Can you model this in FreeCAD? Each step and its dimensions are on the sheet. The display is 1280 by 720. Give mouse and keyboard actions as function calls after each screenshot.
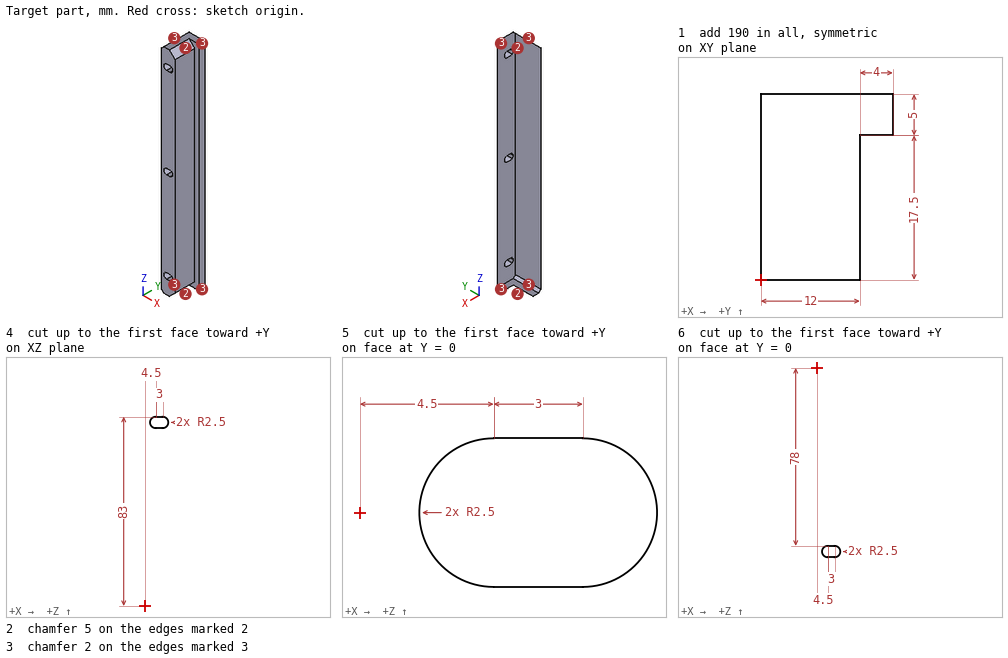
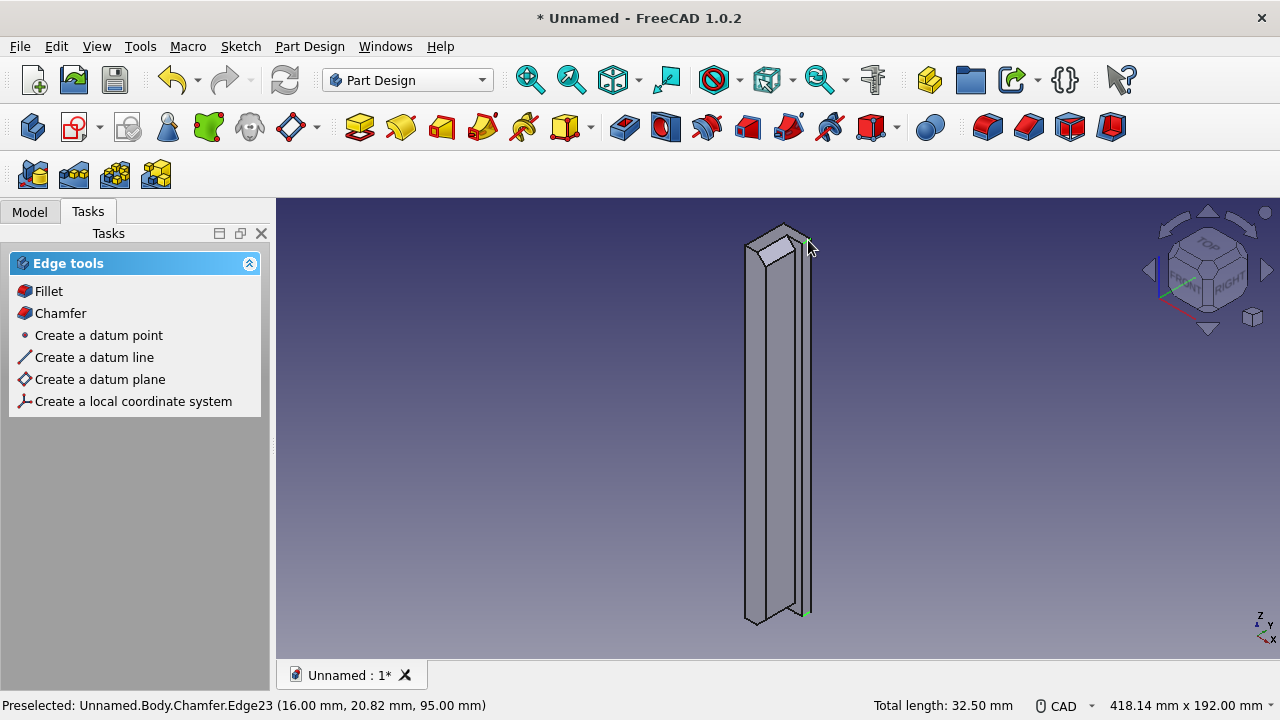
key(2)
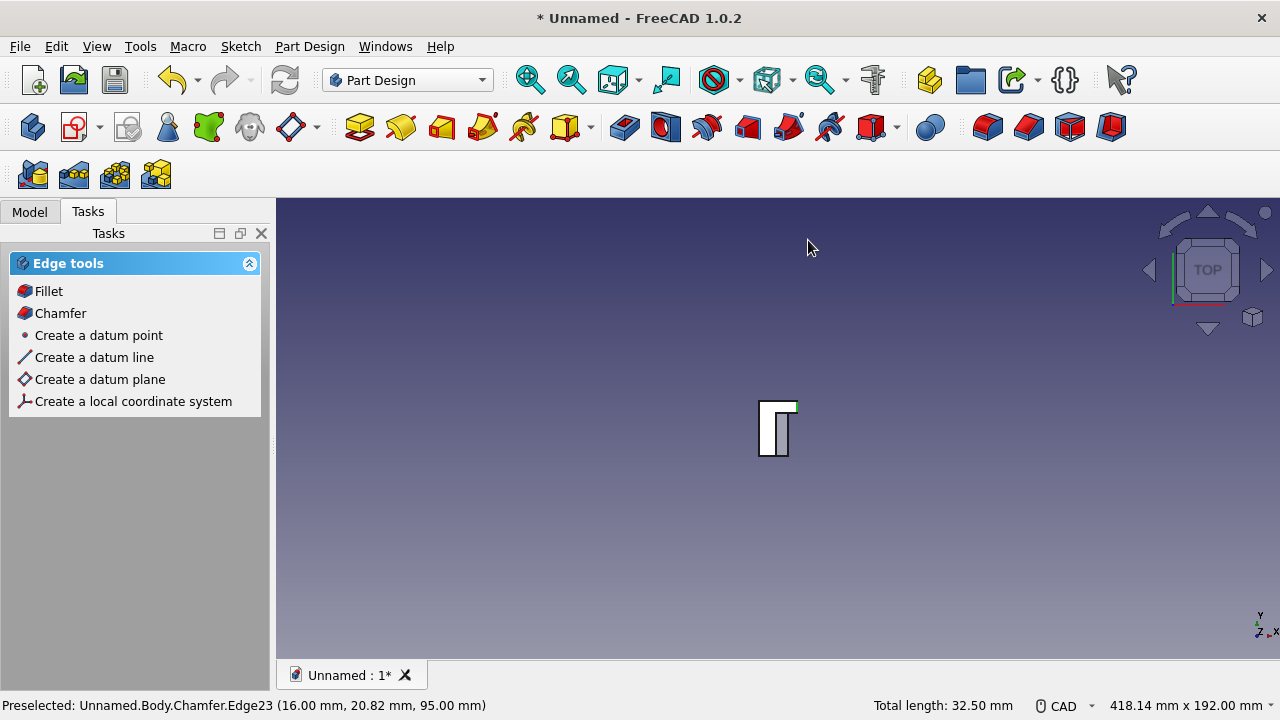
click(531, 80)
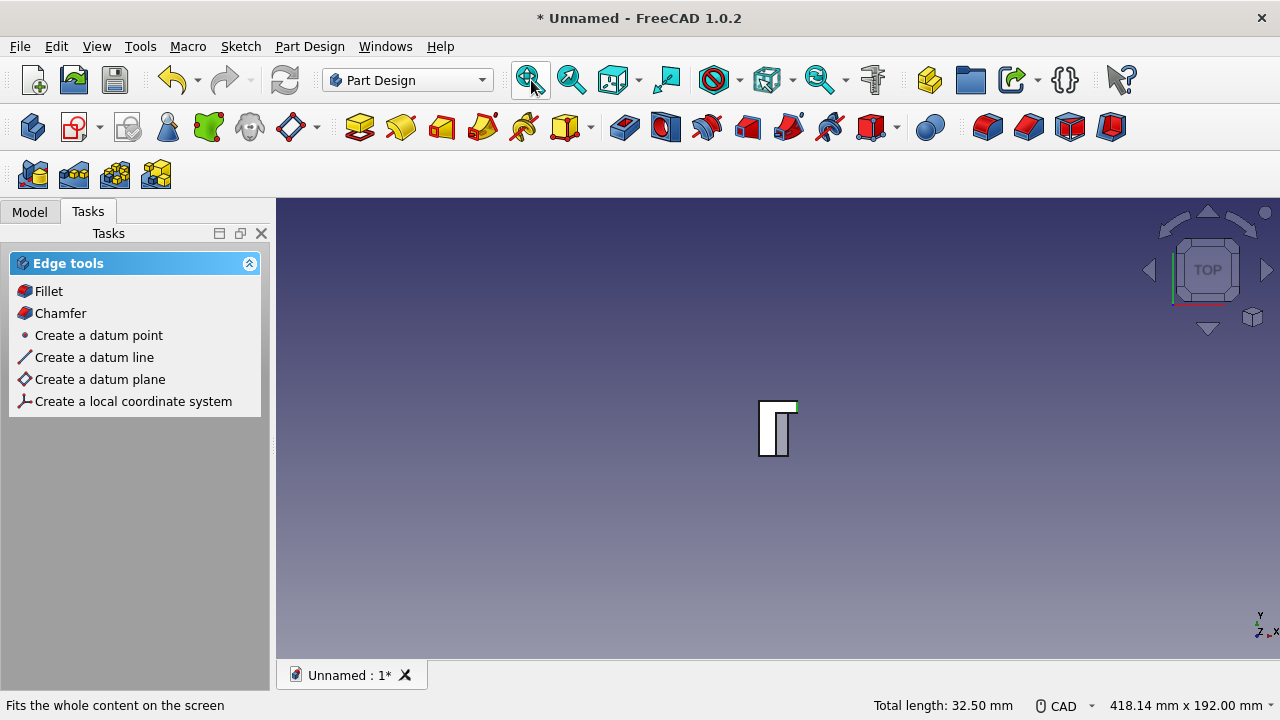
click(759, 427, ctrl)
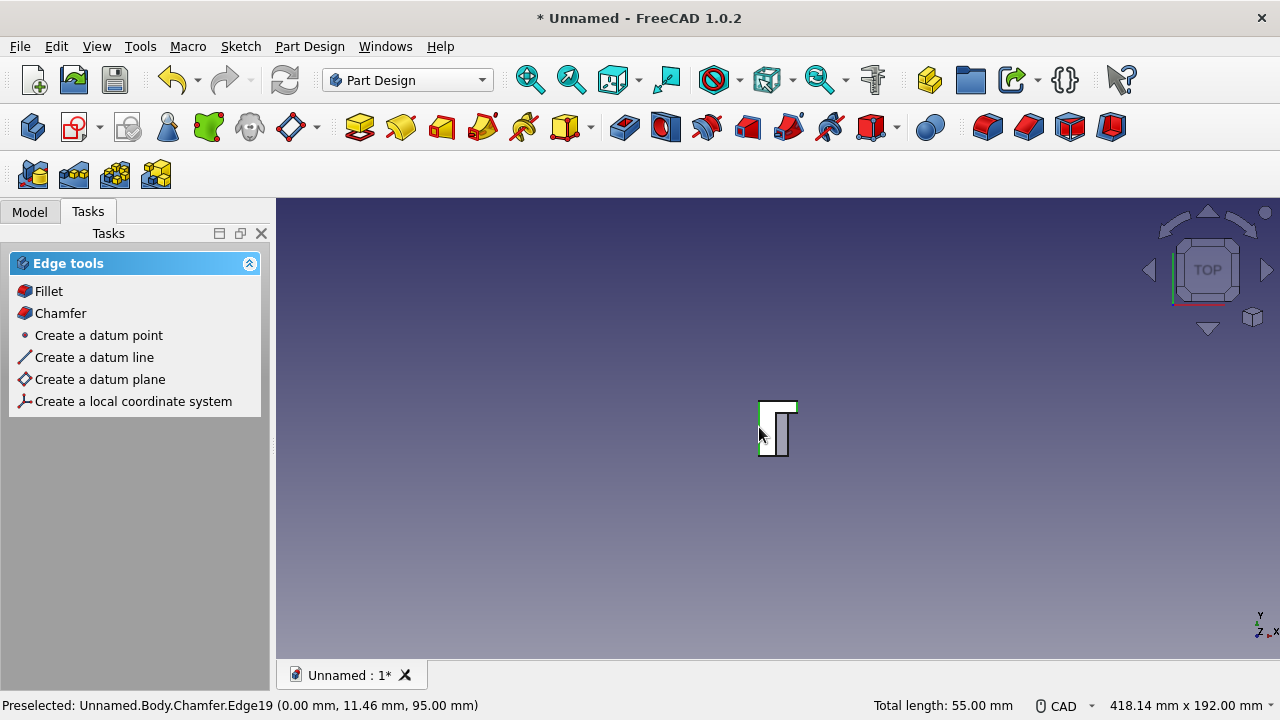
click(1029, 128)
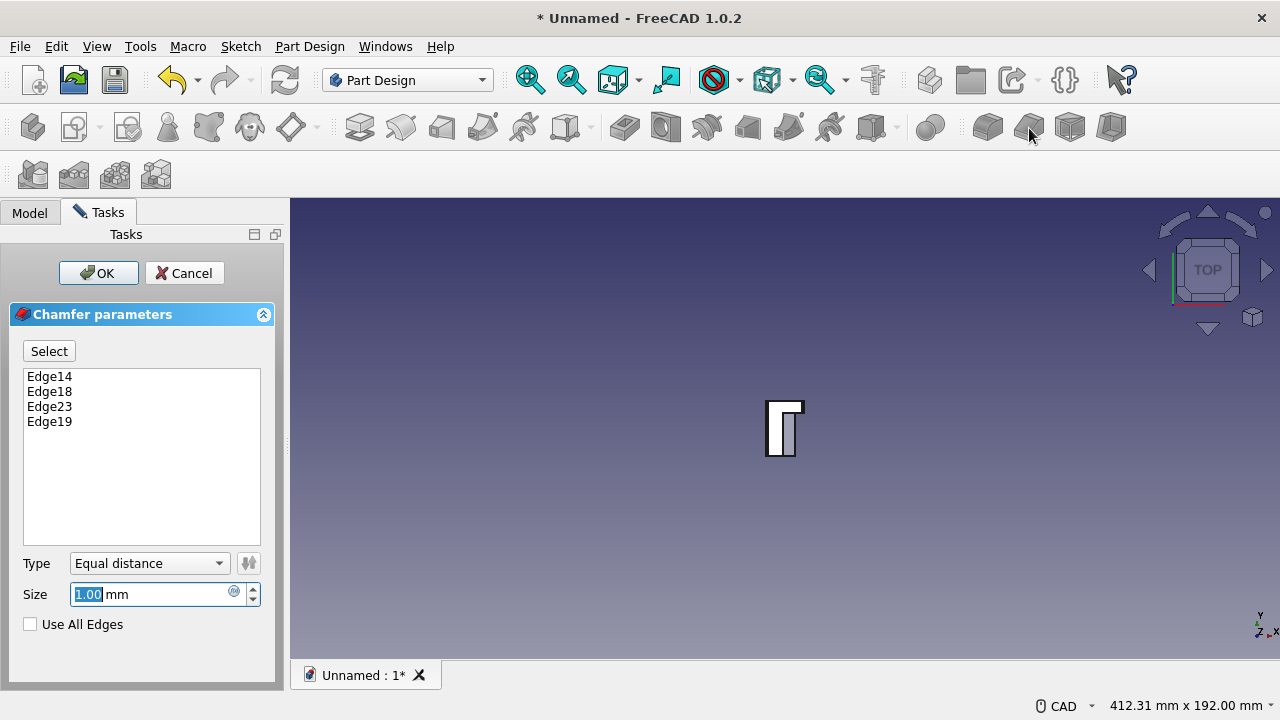
text(2)
key(Tab)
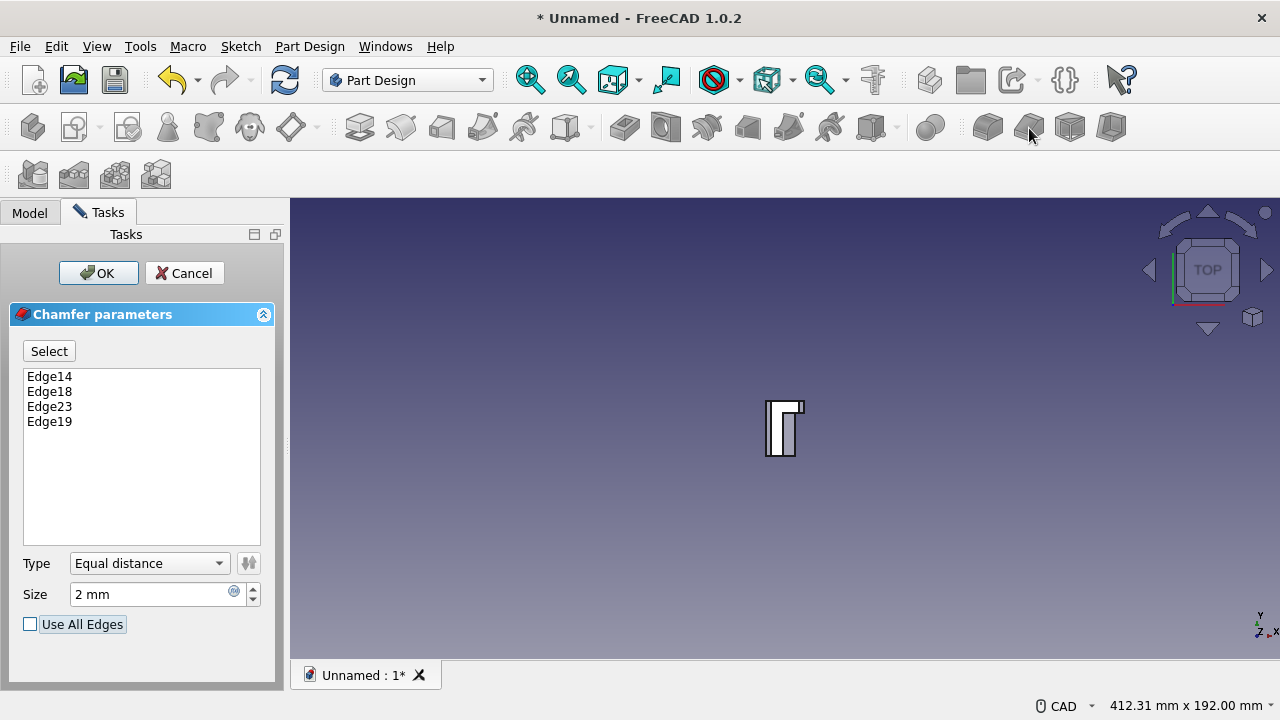
click(99, 273)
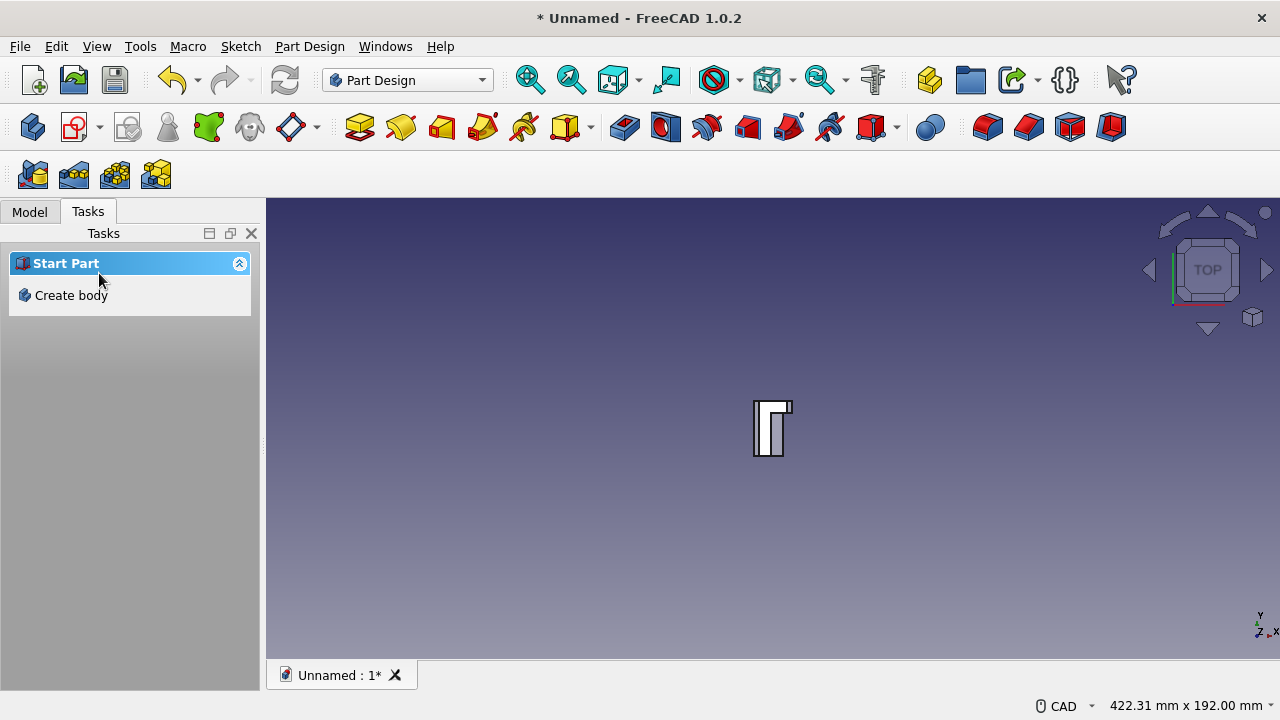
click(531, 80)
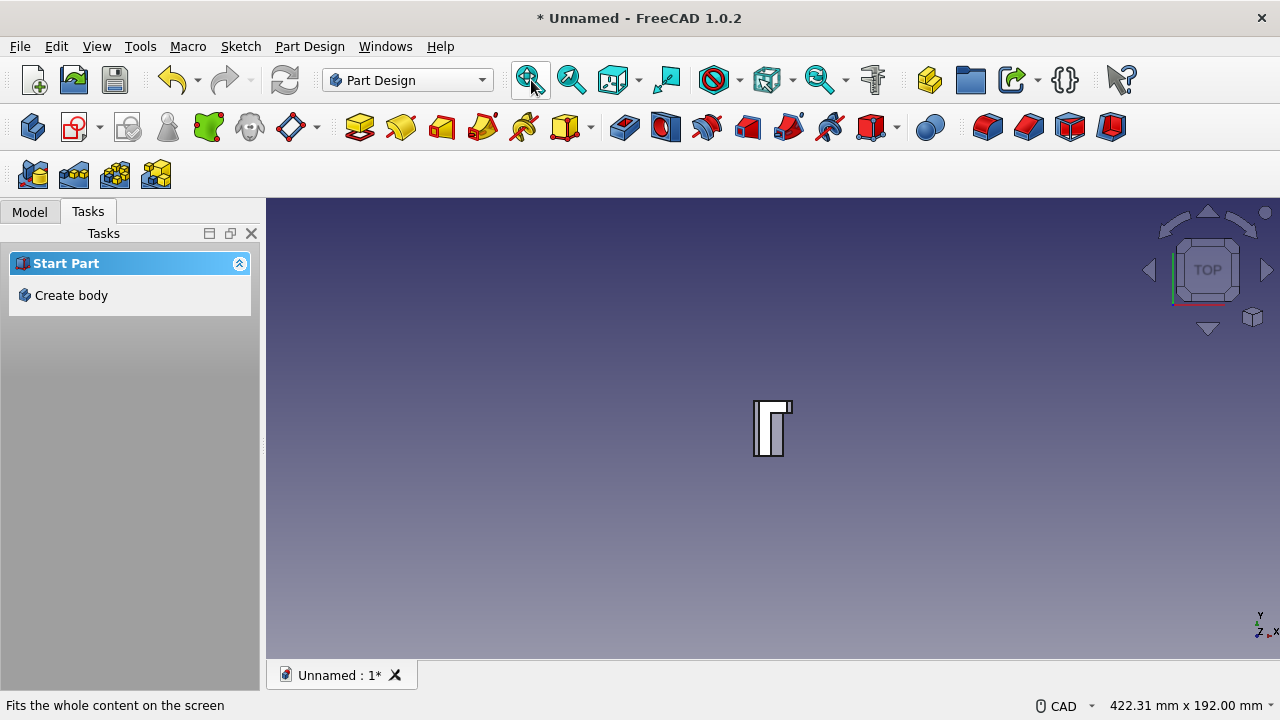
click(74, 128)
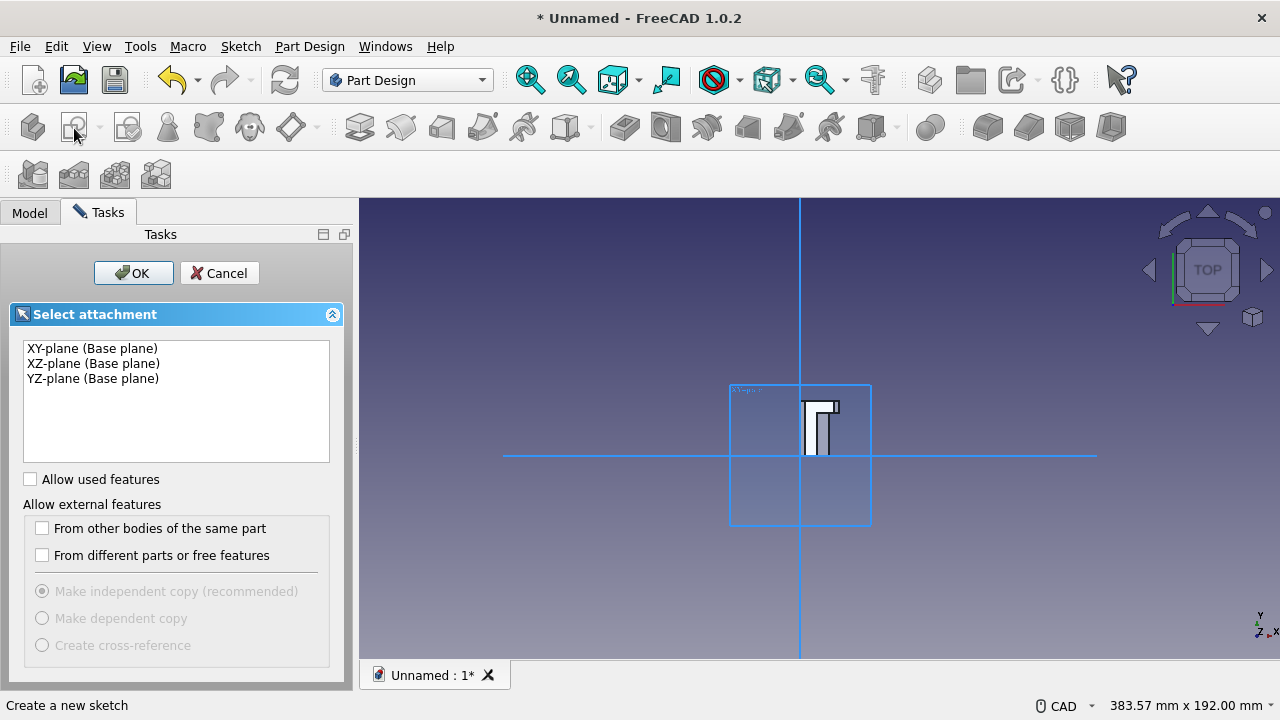
click(84, 364)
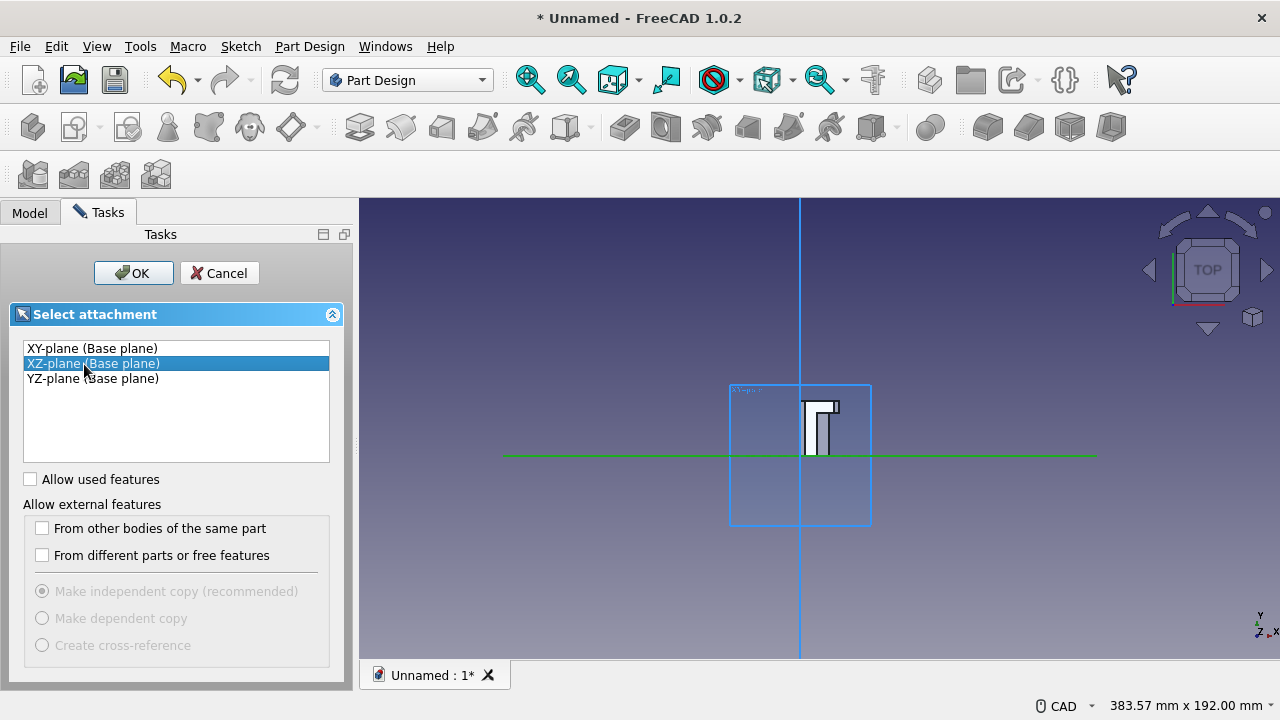
click(134, 273)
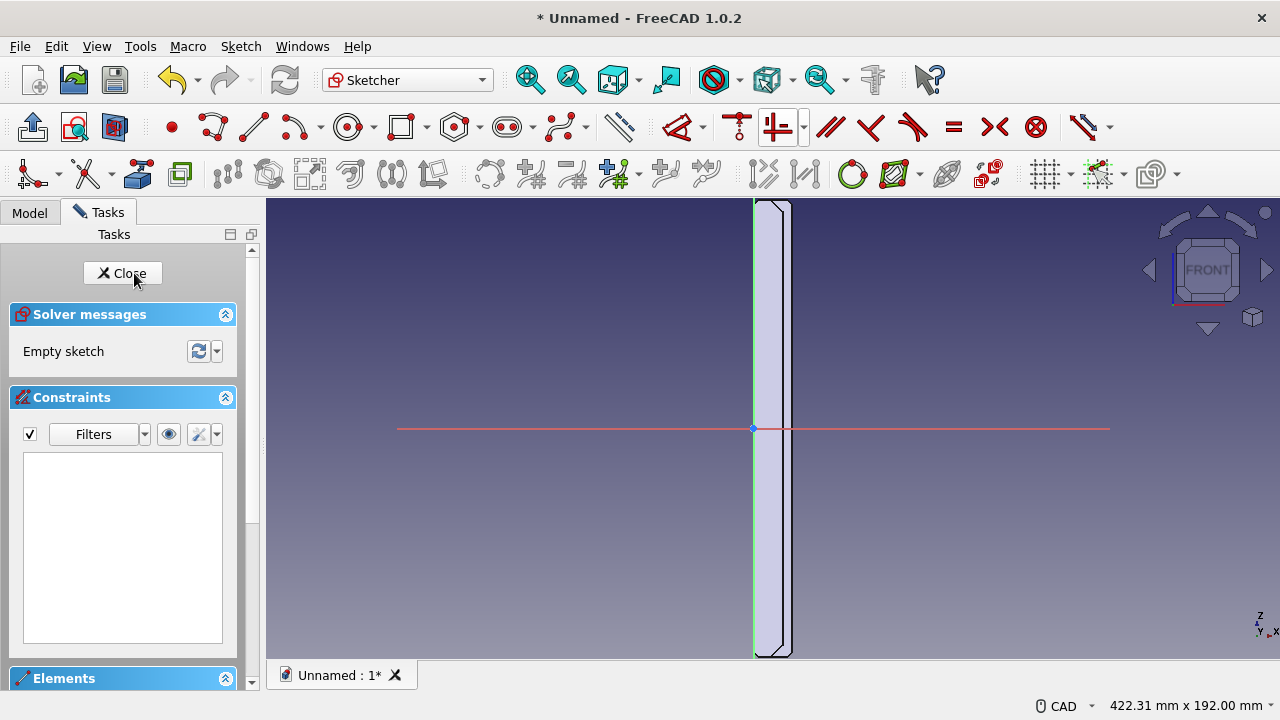
scroll(772, 226, up, 15)